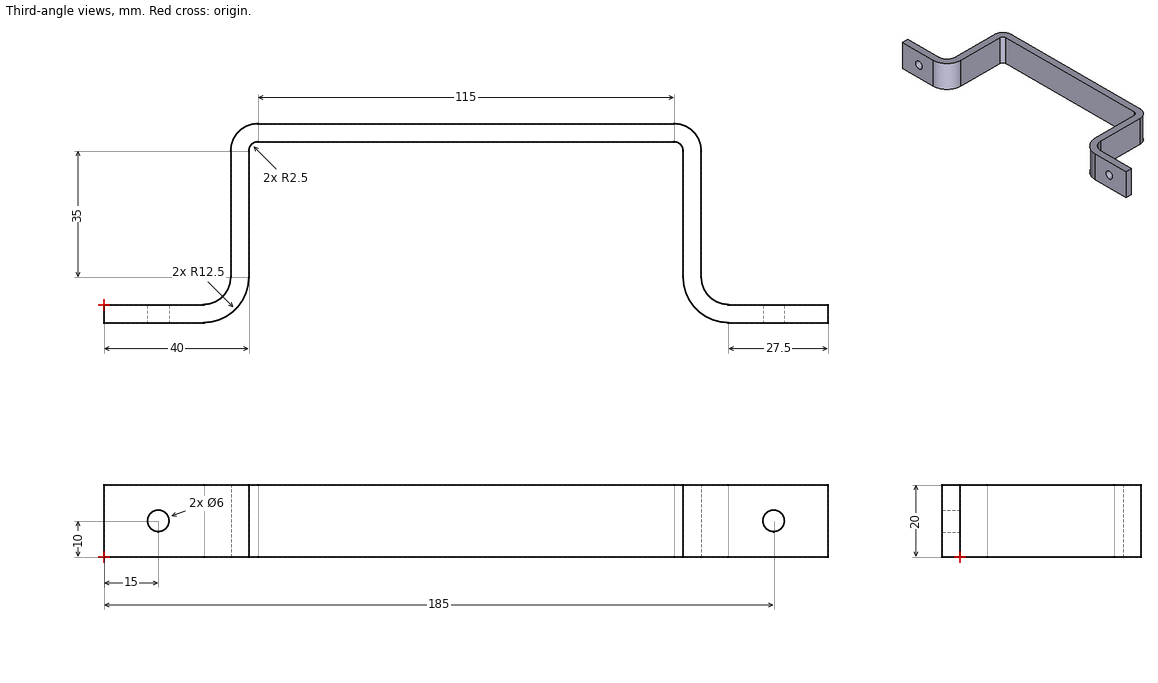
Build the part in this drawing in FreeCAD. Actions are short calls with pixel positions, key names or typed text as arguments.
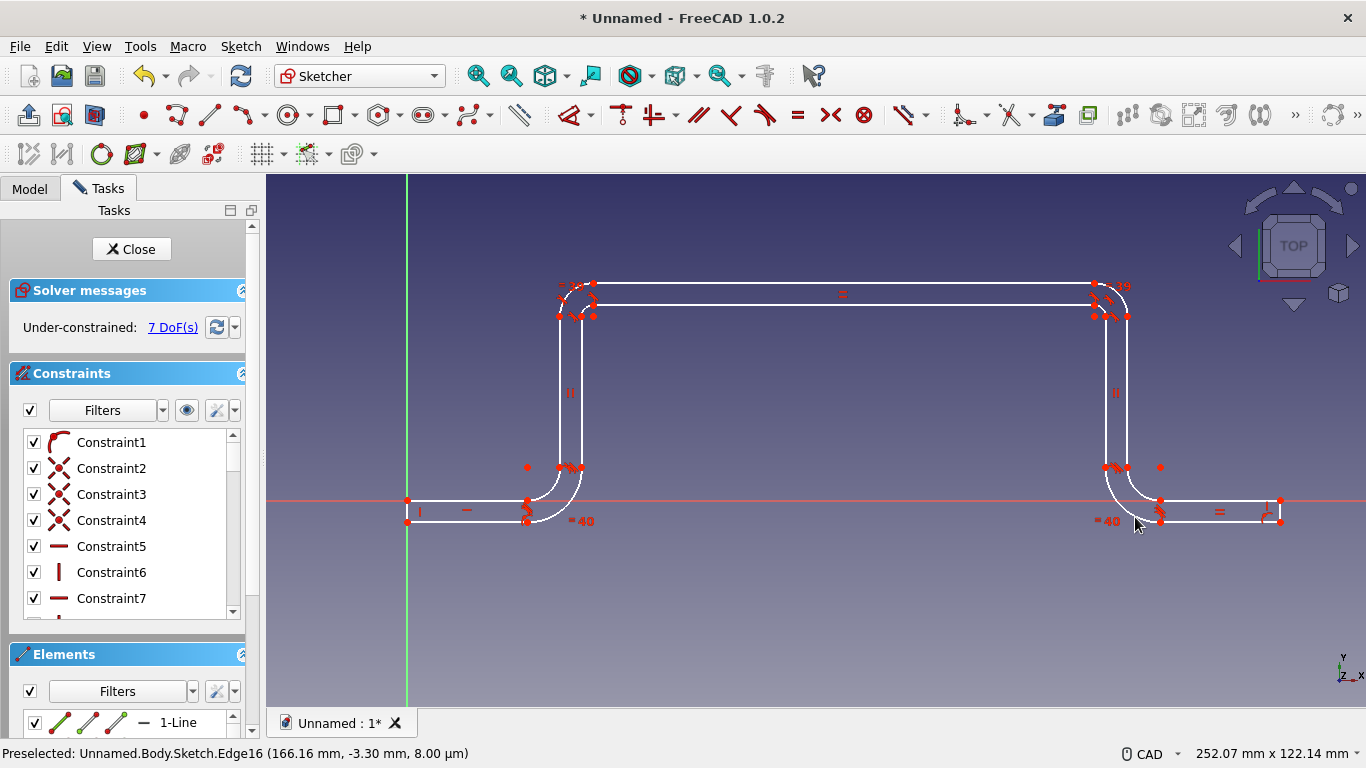
click(1131, 483)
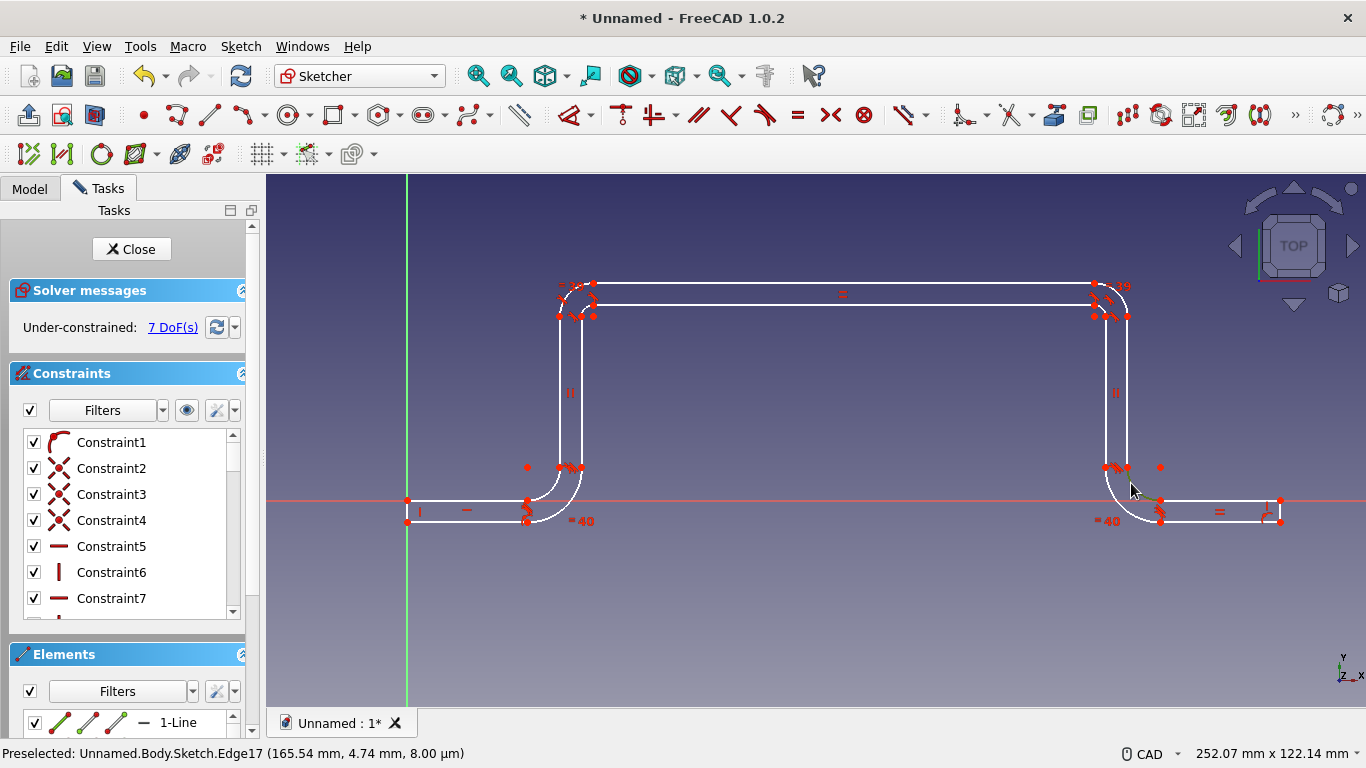
scroll(1124, 301, up, 4)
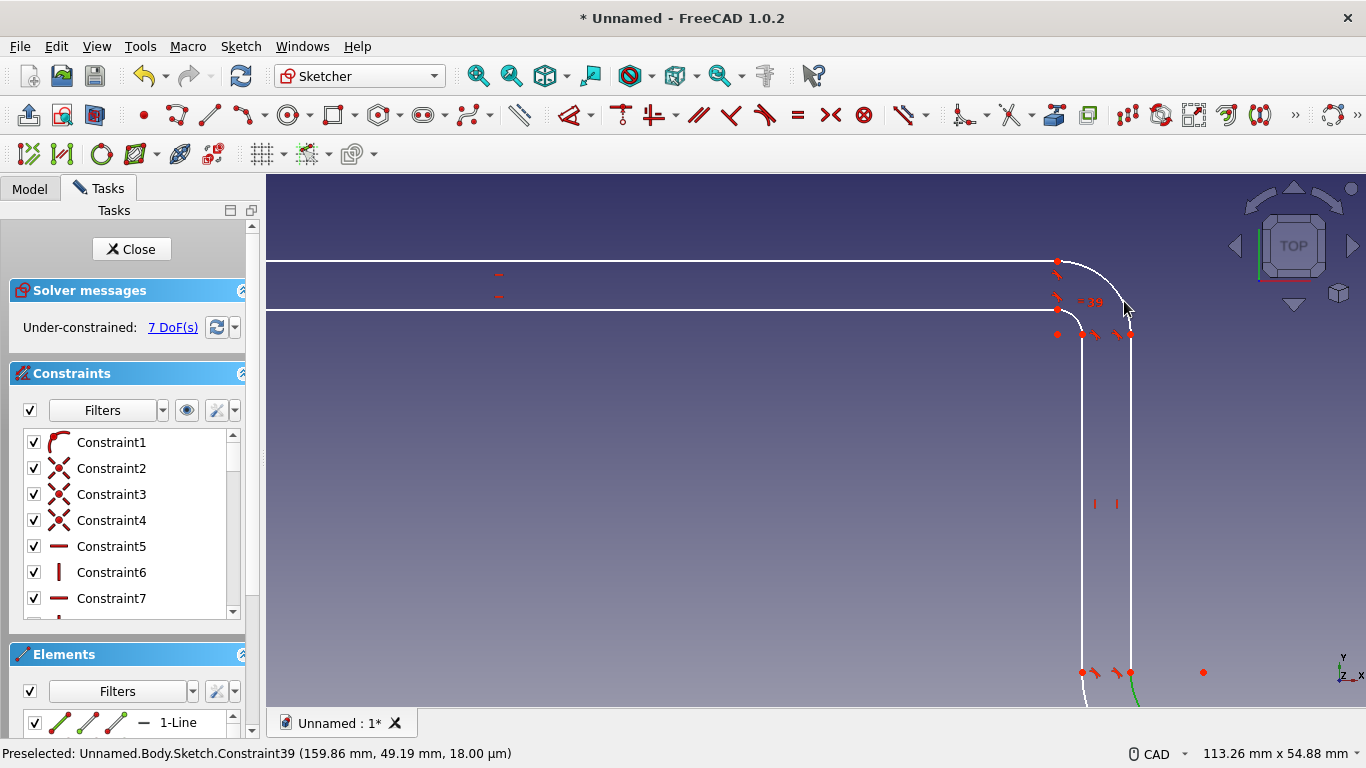
click(1123, 302)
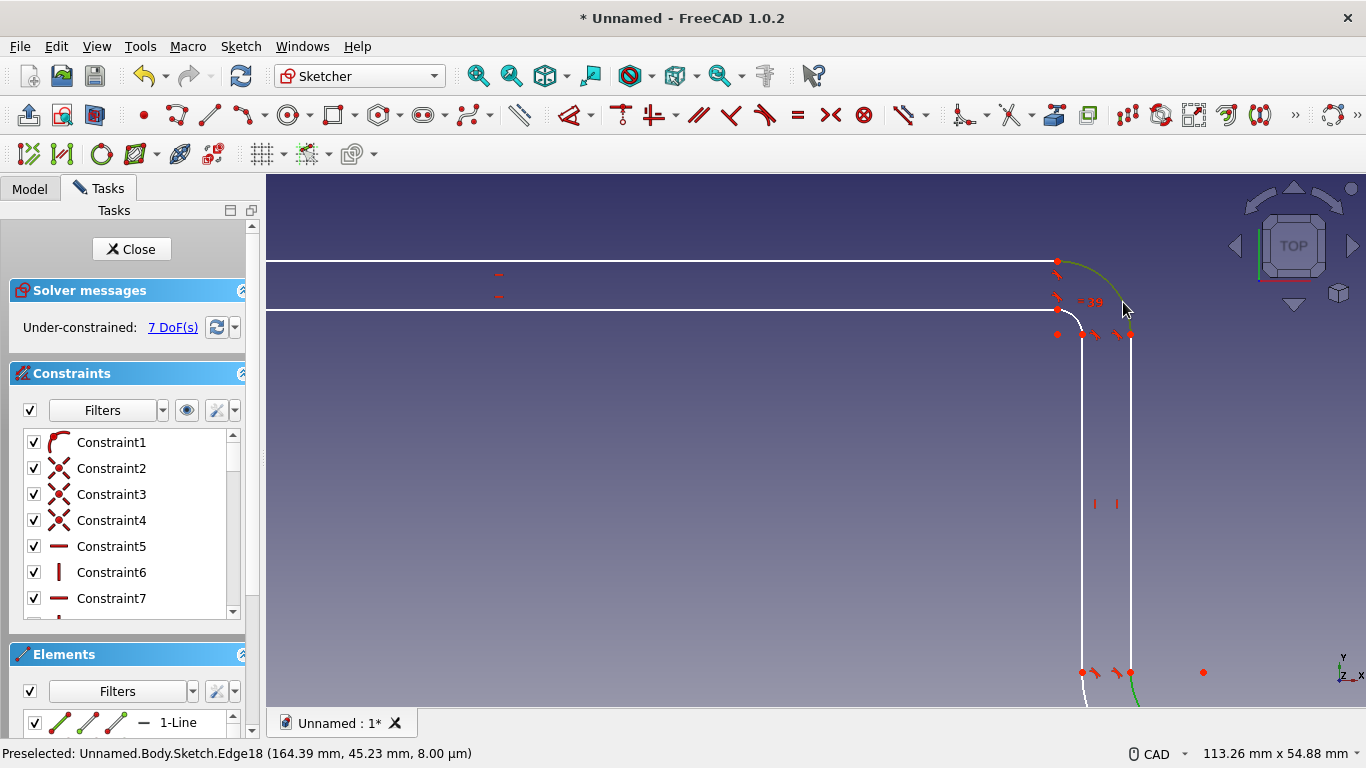
click(798, 116)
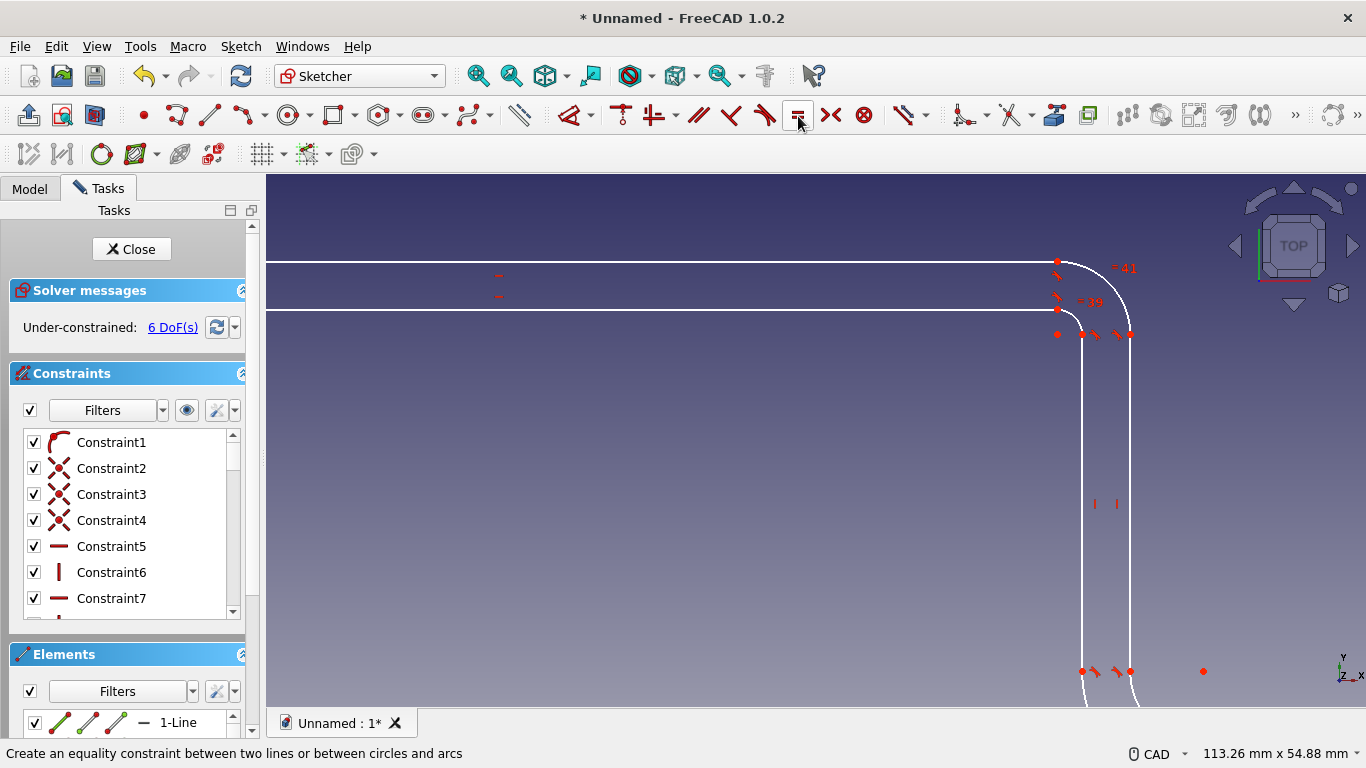
scroll(854, 403, down, 6)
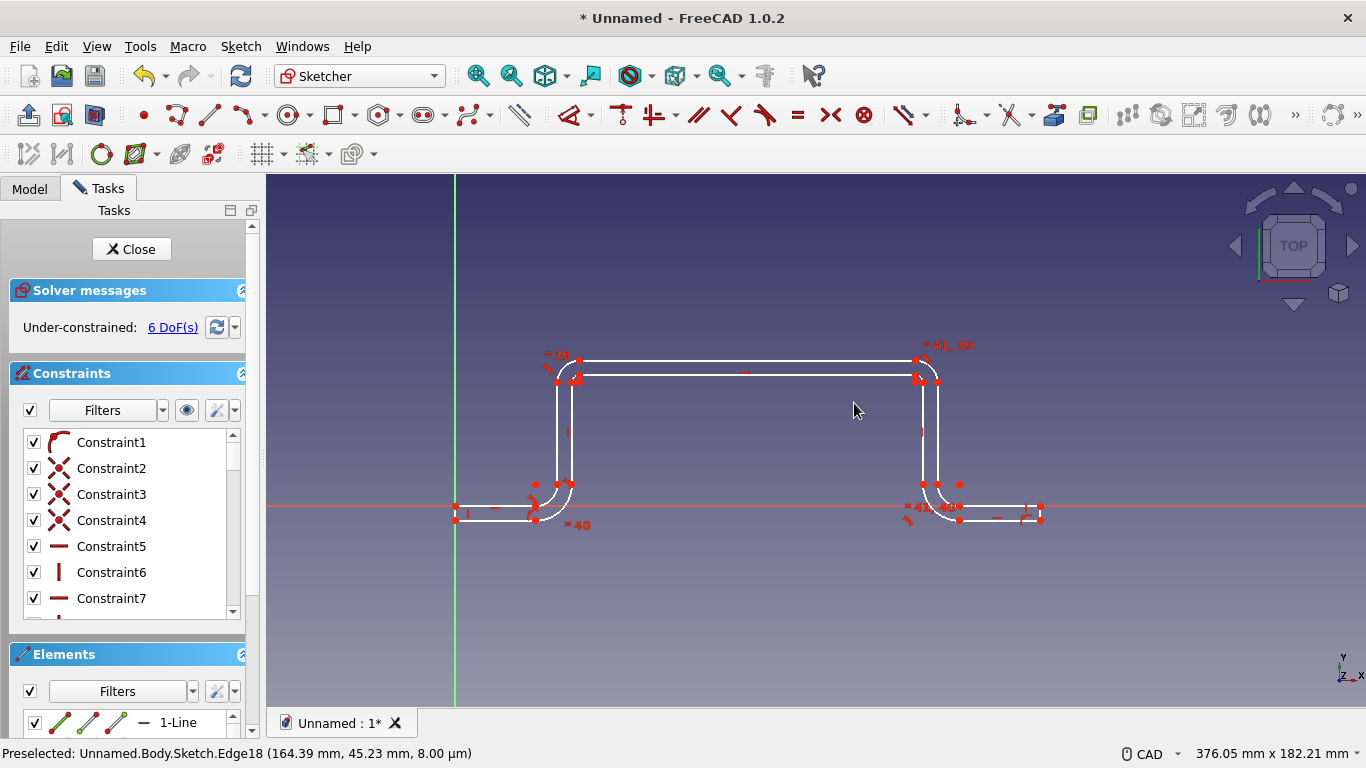
scroll(552, 517, up, 2)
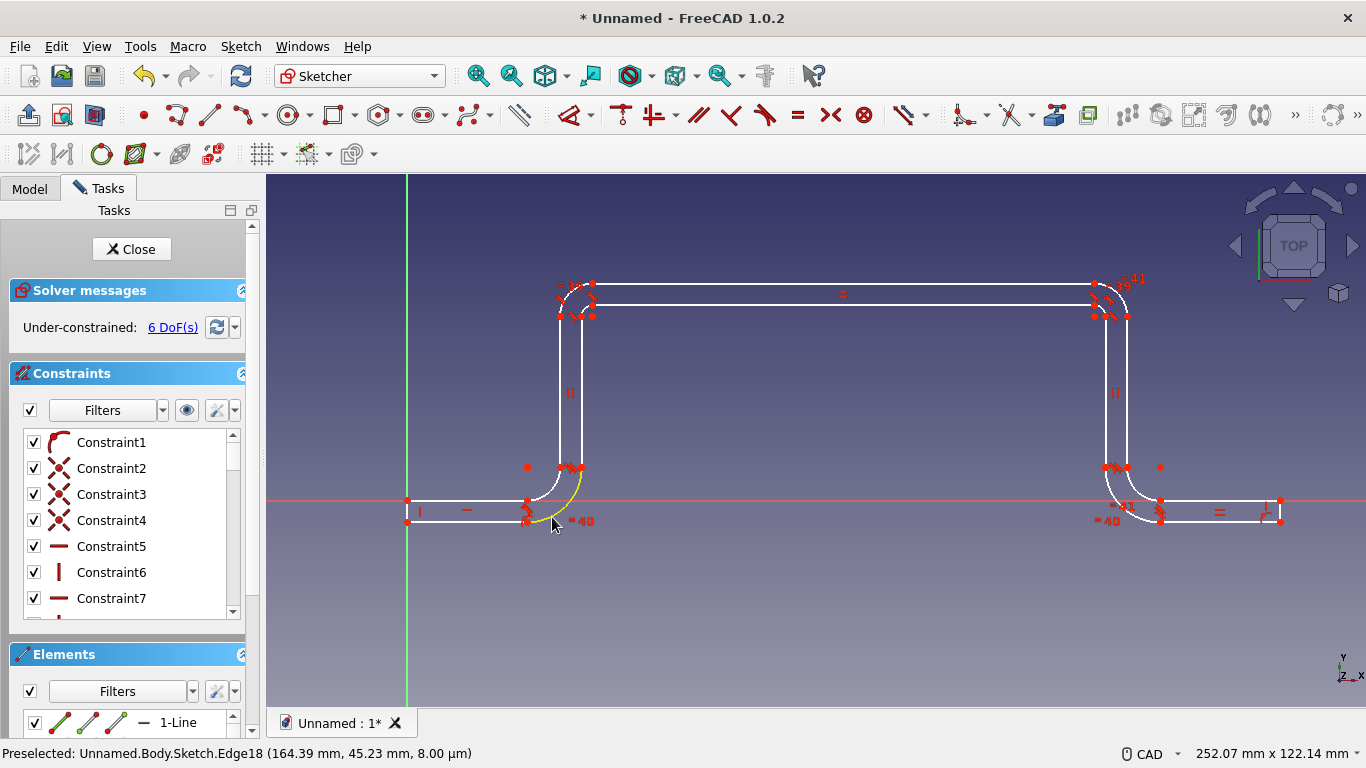
click(552, 516)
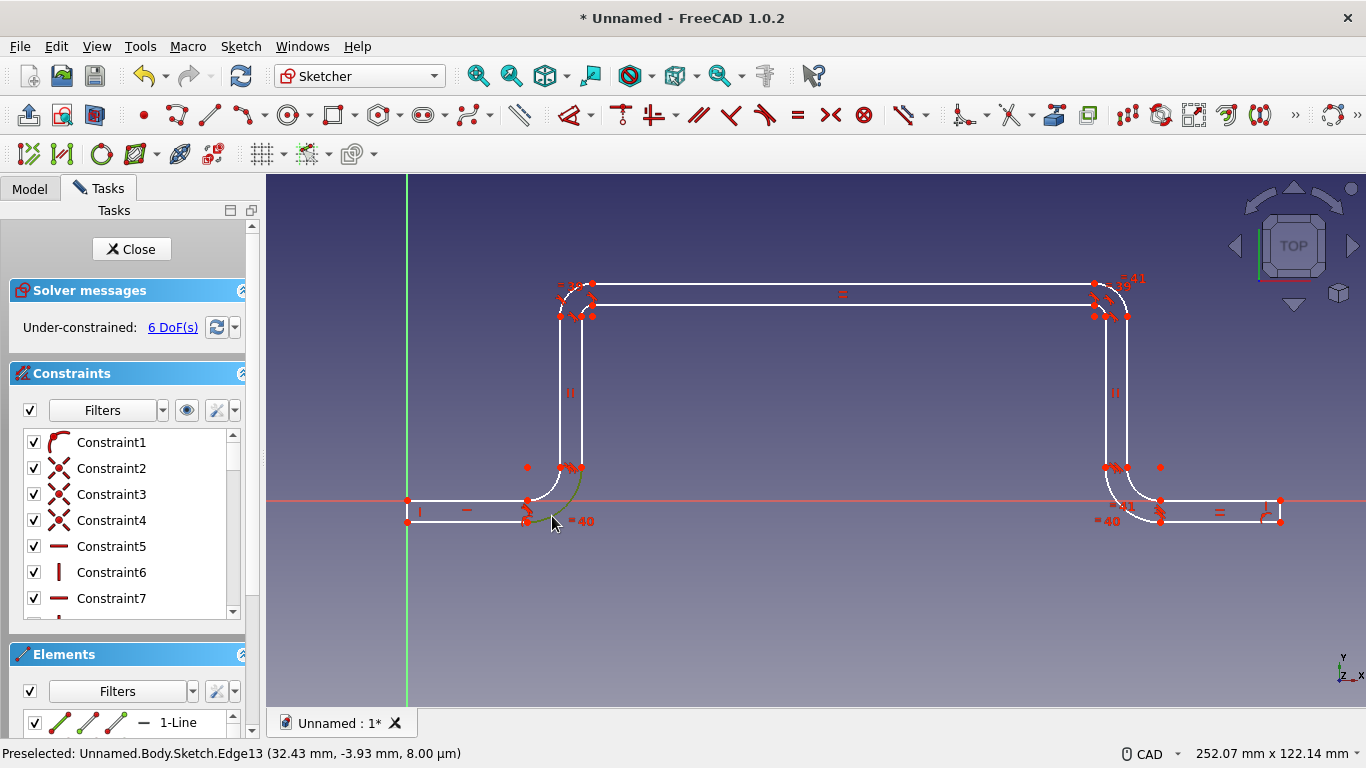
key(k)
key(r)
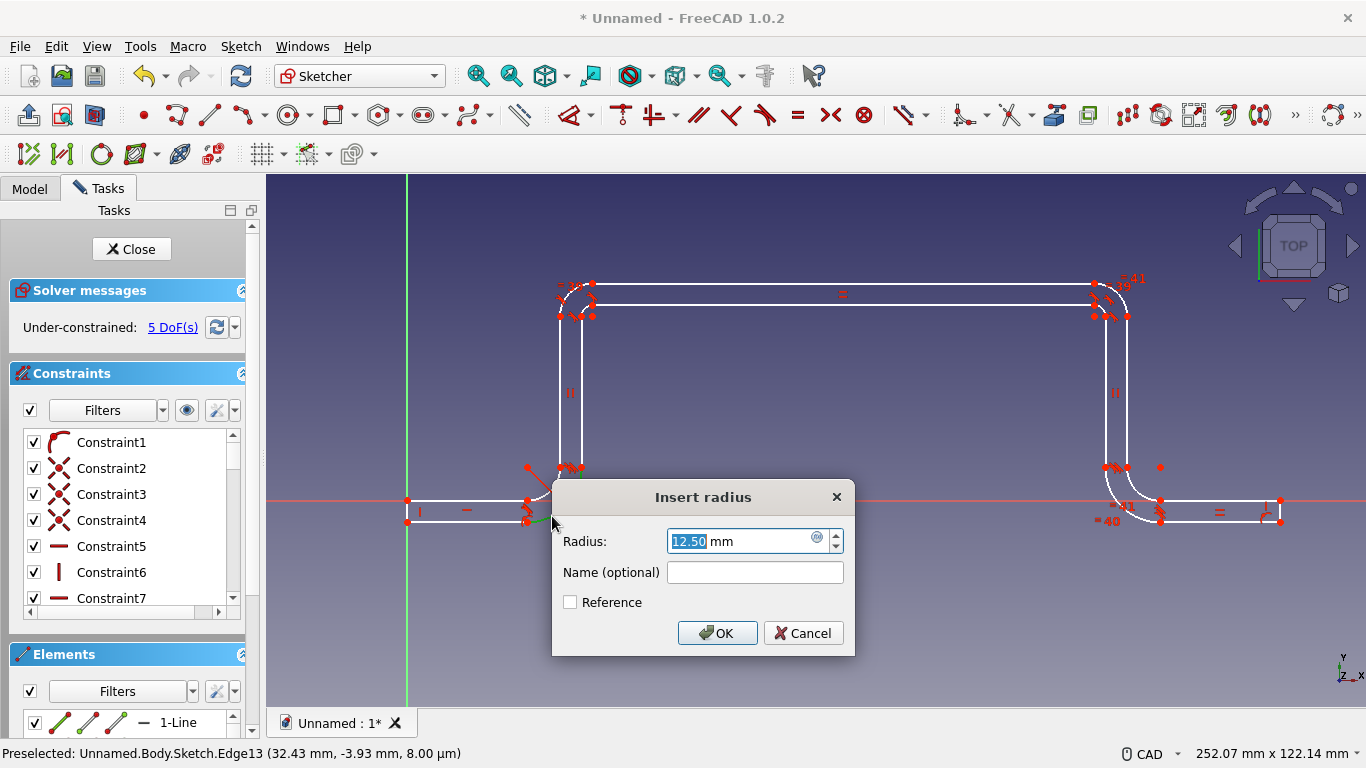
text(12.5)
key(Return)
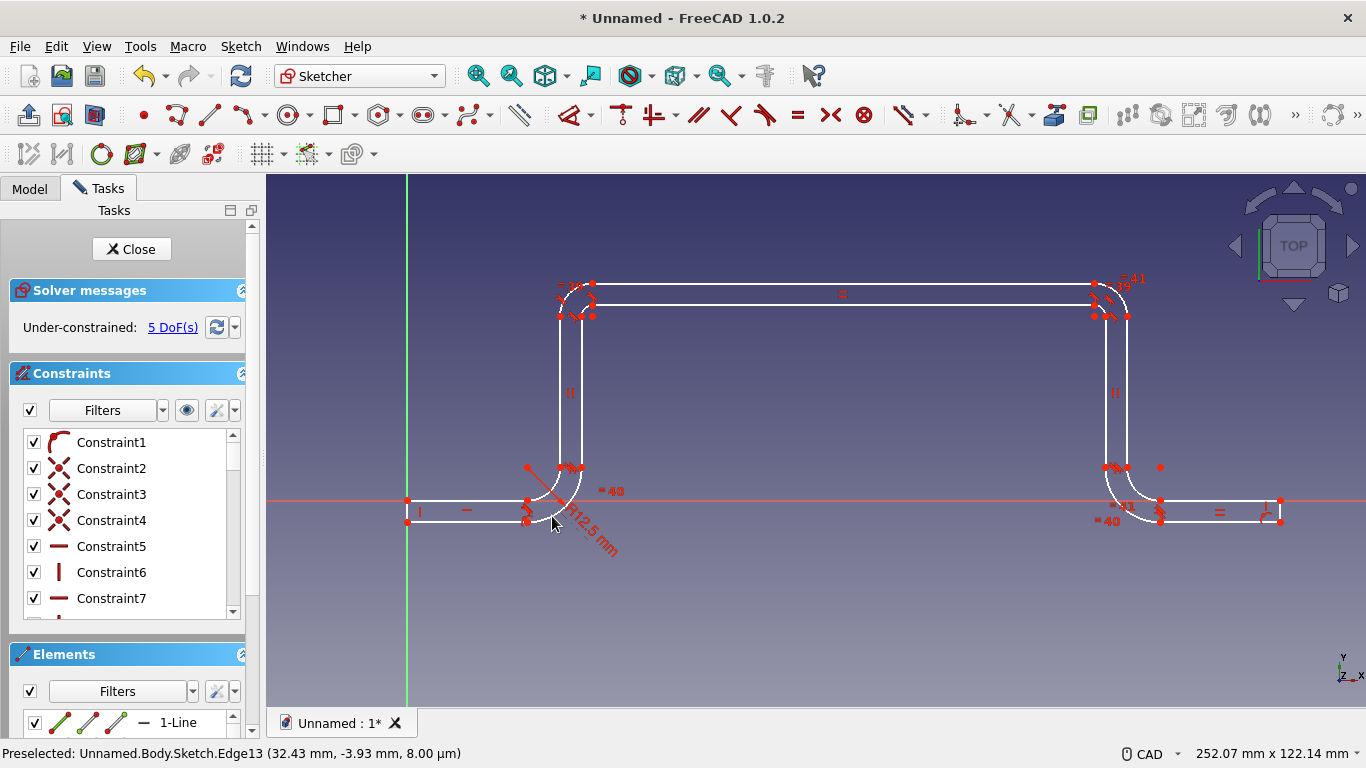
scroll(585, 308, up, 7)